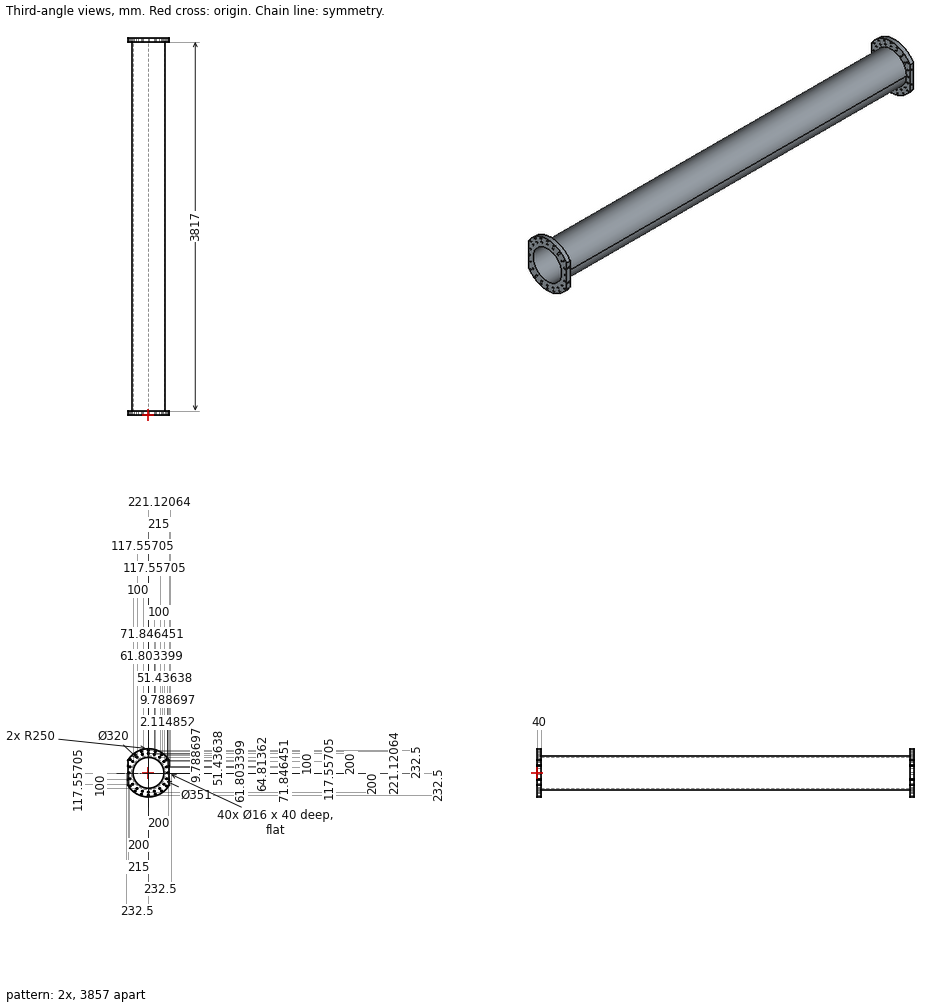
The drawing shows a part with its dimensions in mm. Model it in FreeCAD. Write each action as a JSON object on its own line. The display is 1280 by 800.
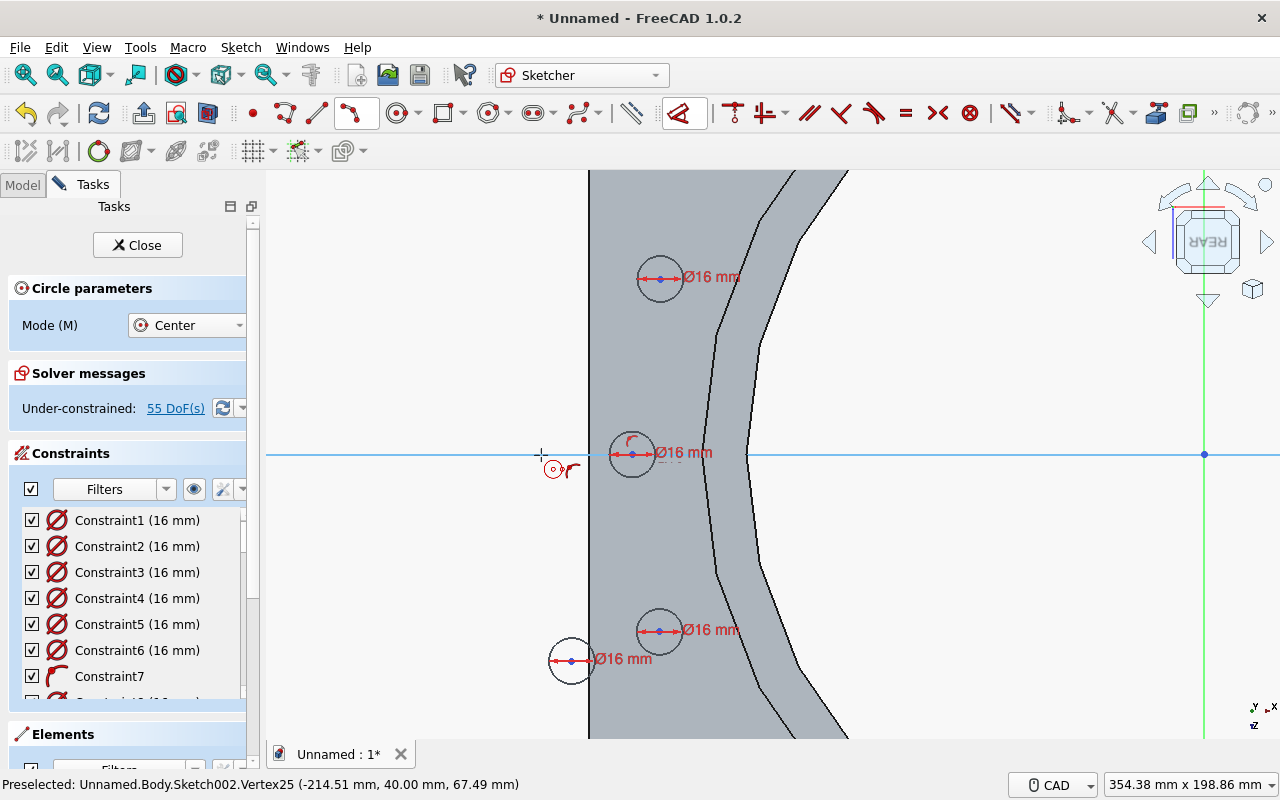
{"action": "left_click", "coordinate": [539, 455]}
{"action": "mouse_move", "coordinate": [555, 438]}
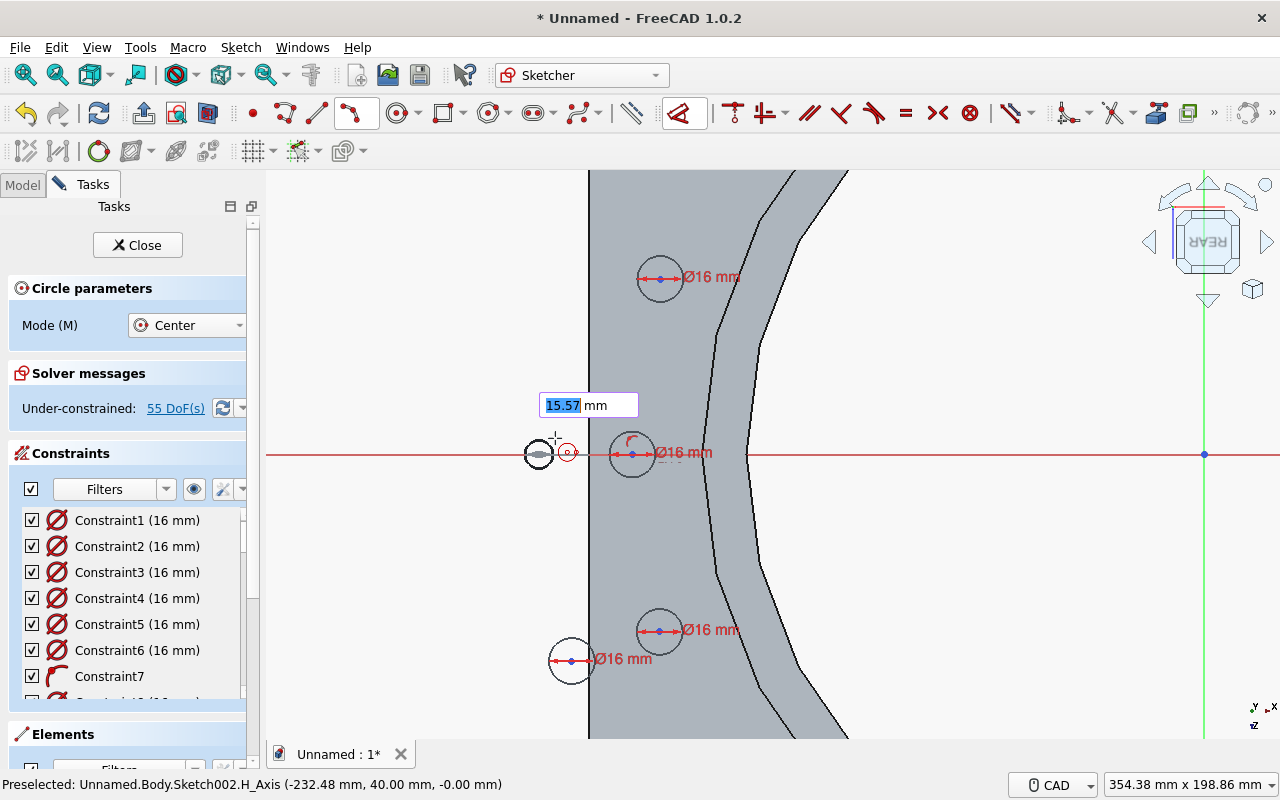
{"action": "type", "text": "16"}
{"action": "key", "text": "Return"}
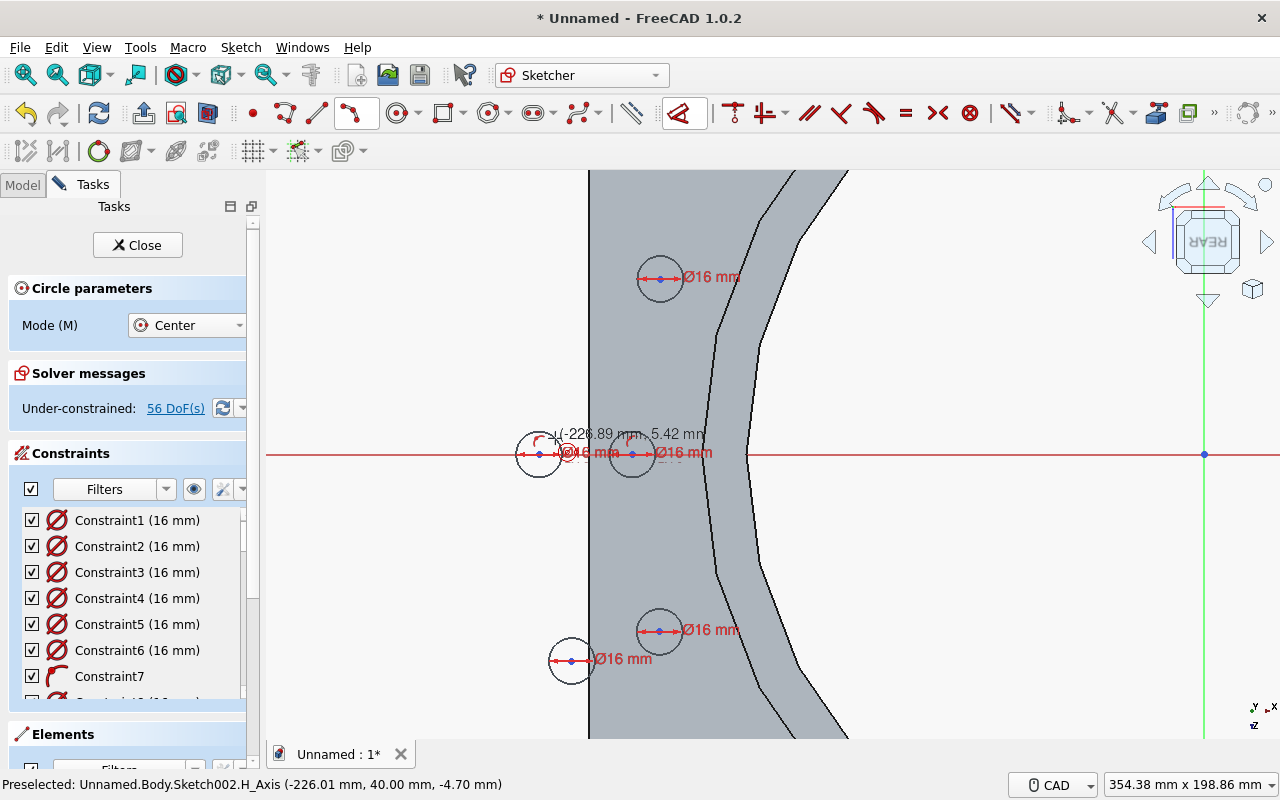
{"action": "left_click", "coordinate": [572, 249]}
{"action": "mouse_move", "coordinate": [588, 233]}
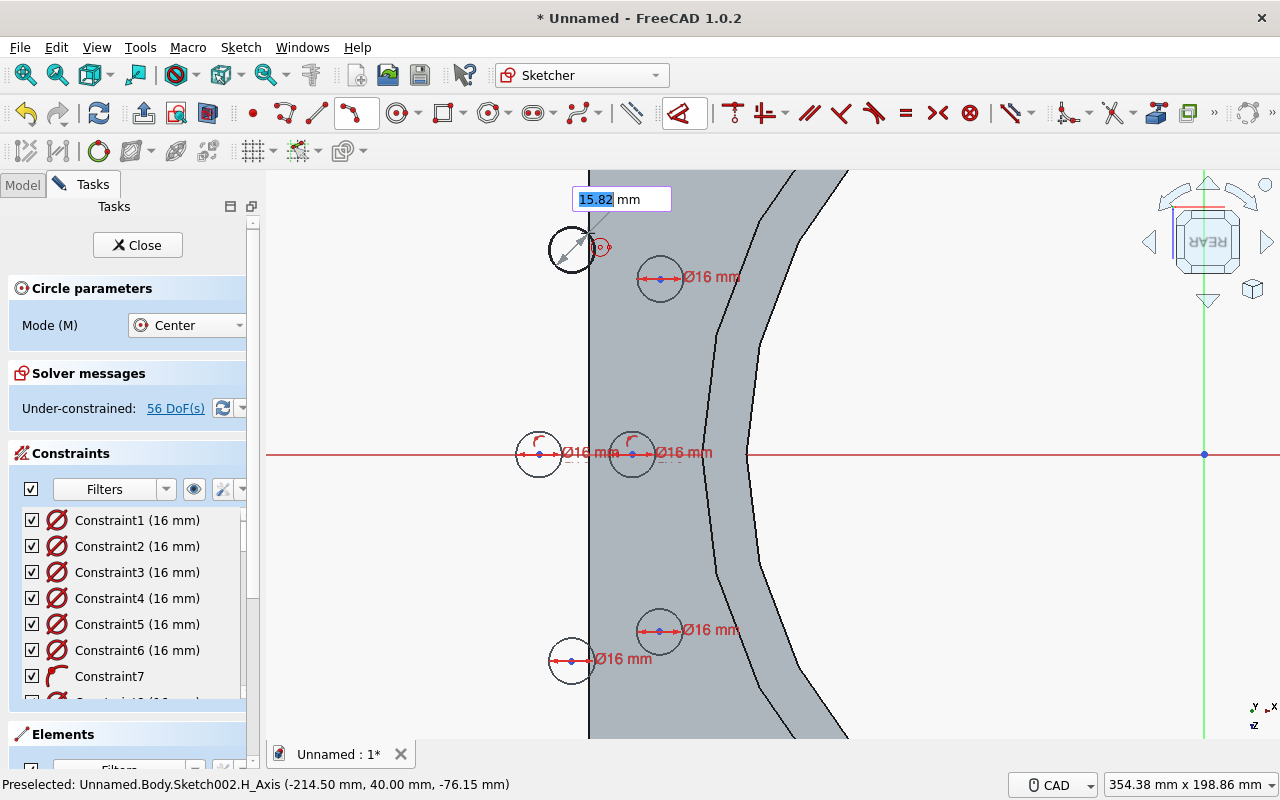
{"action": "type", "text": "16"}
{"action": "key", "text": "Return"}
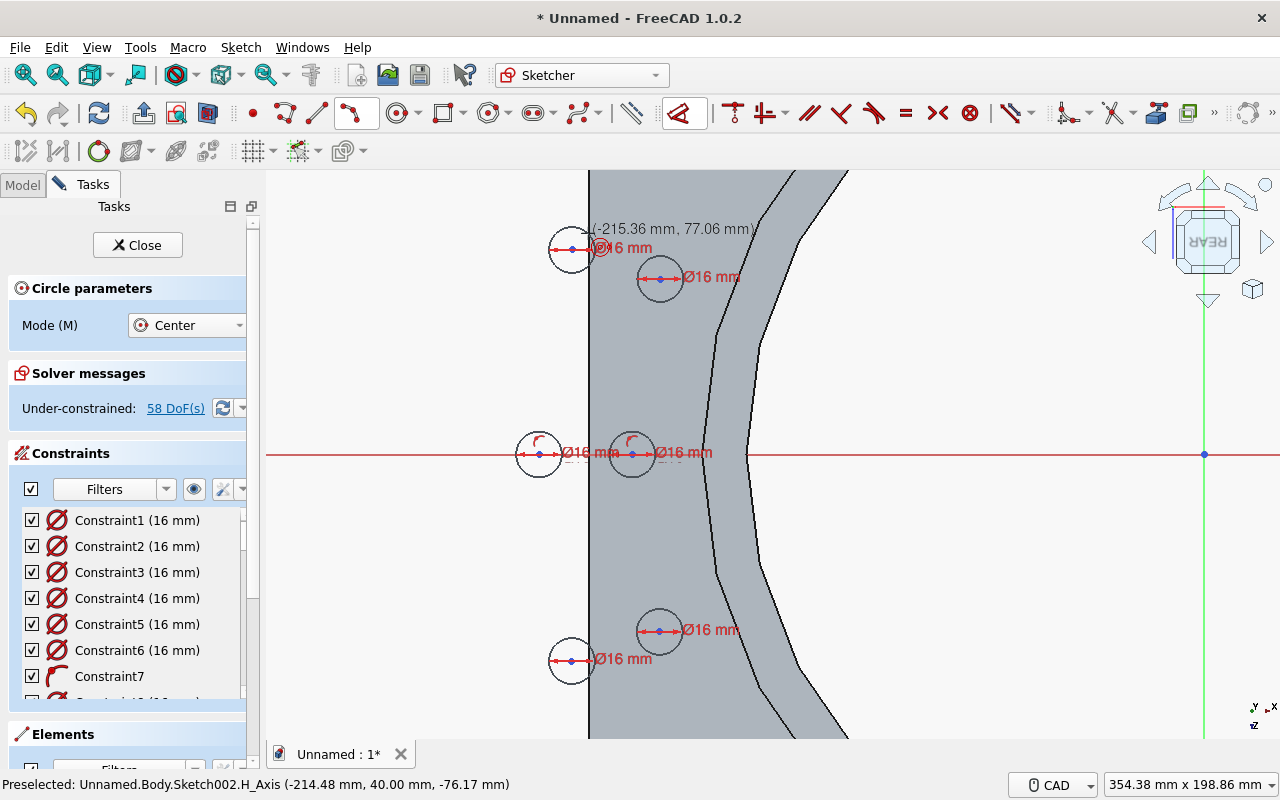
{"action": "scroll", "coordinate": [541, 454], "scroll_direction": "down", "scroll_amount": 7}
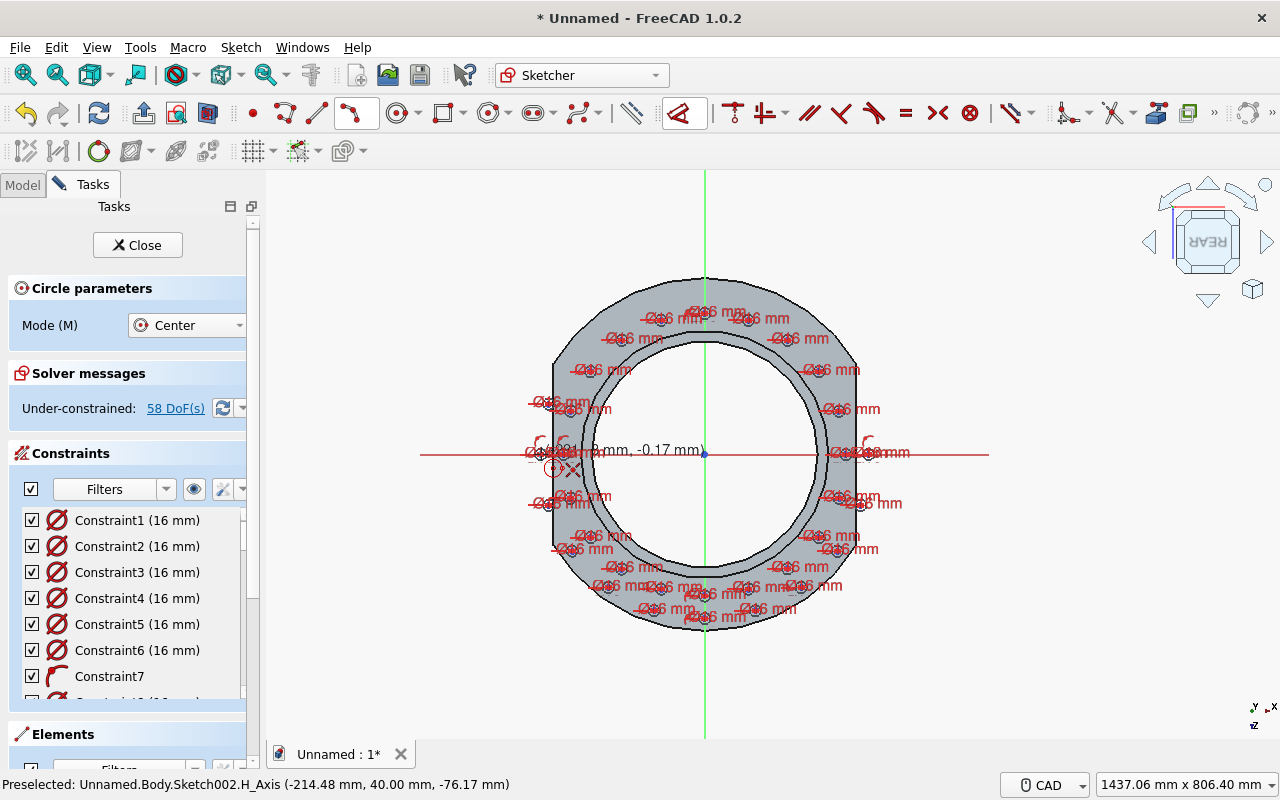
{"action": "scroll", "coordinate": [572, 358], "scroll_direction": "up", "scroll_amount": 7}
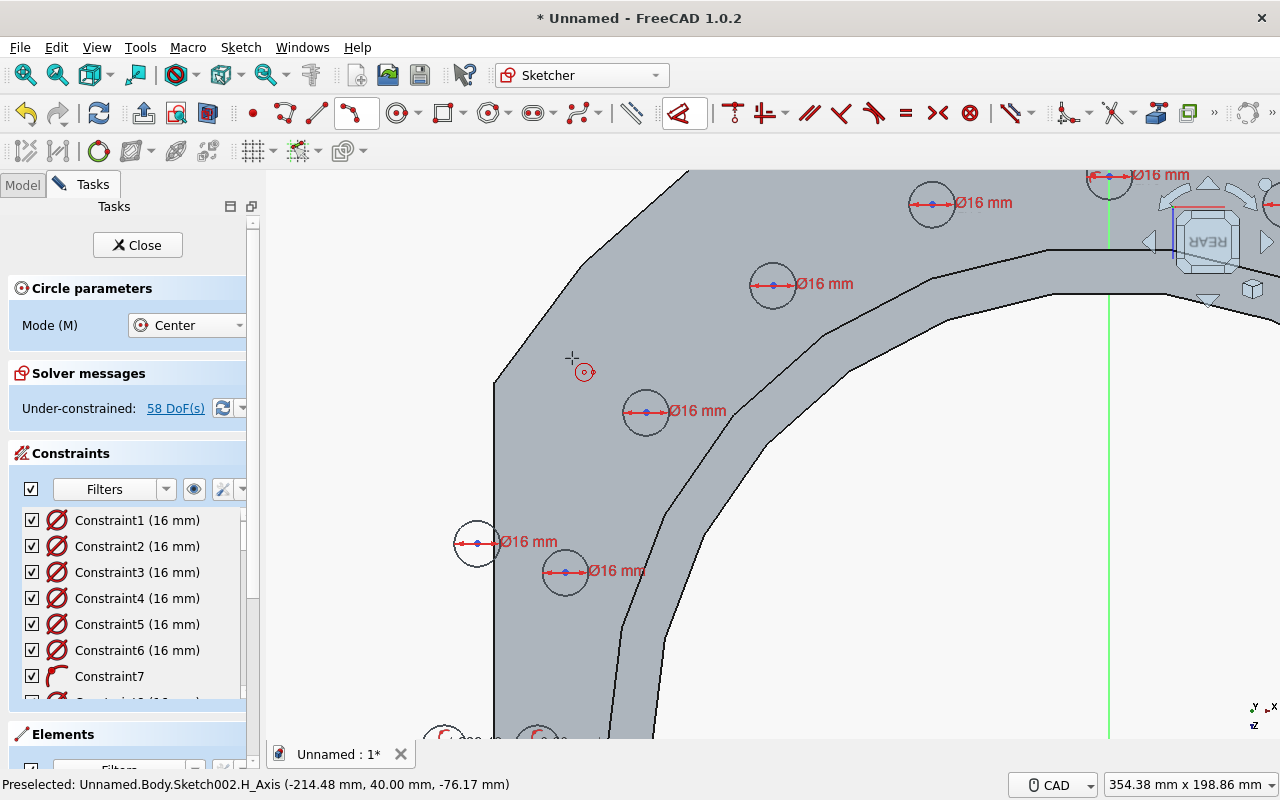
{"action": "left_click", "coordinate": [571, 357]}
{"action": "mouse_move", "coordinate": [587, 341]}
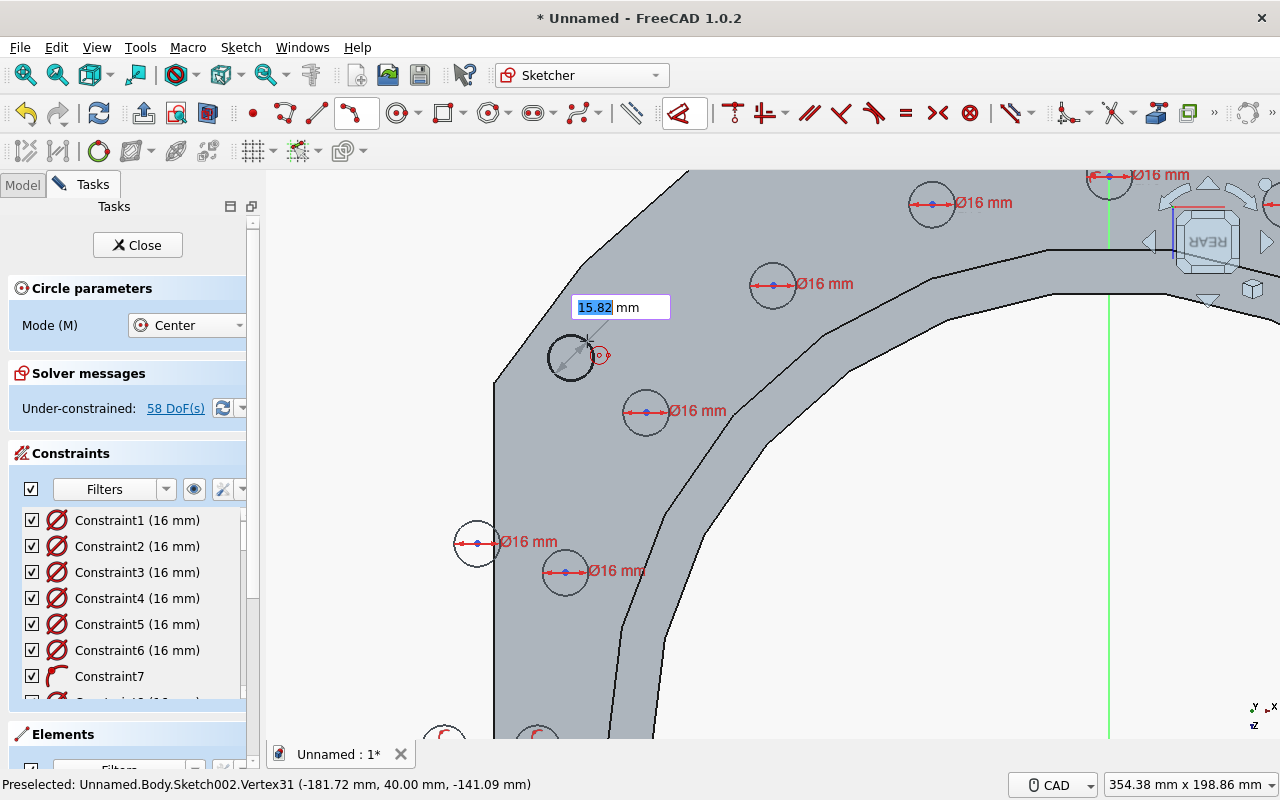
{"action": "type", "text": "16"}
{"action": "key", "text": "Return"}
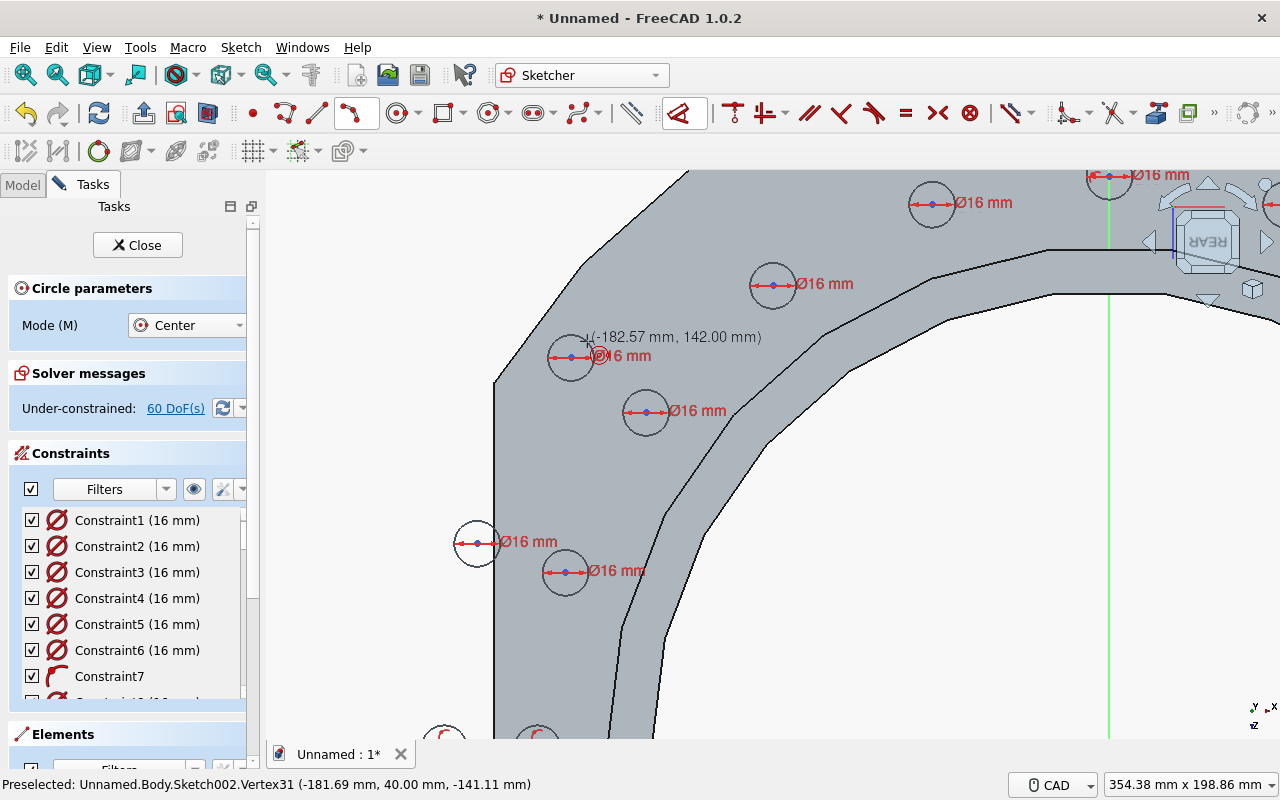
{"action": "left_click", "coordinate": [718, 210]}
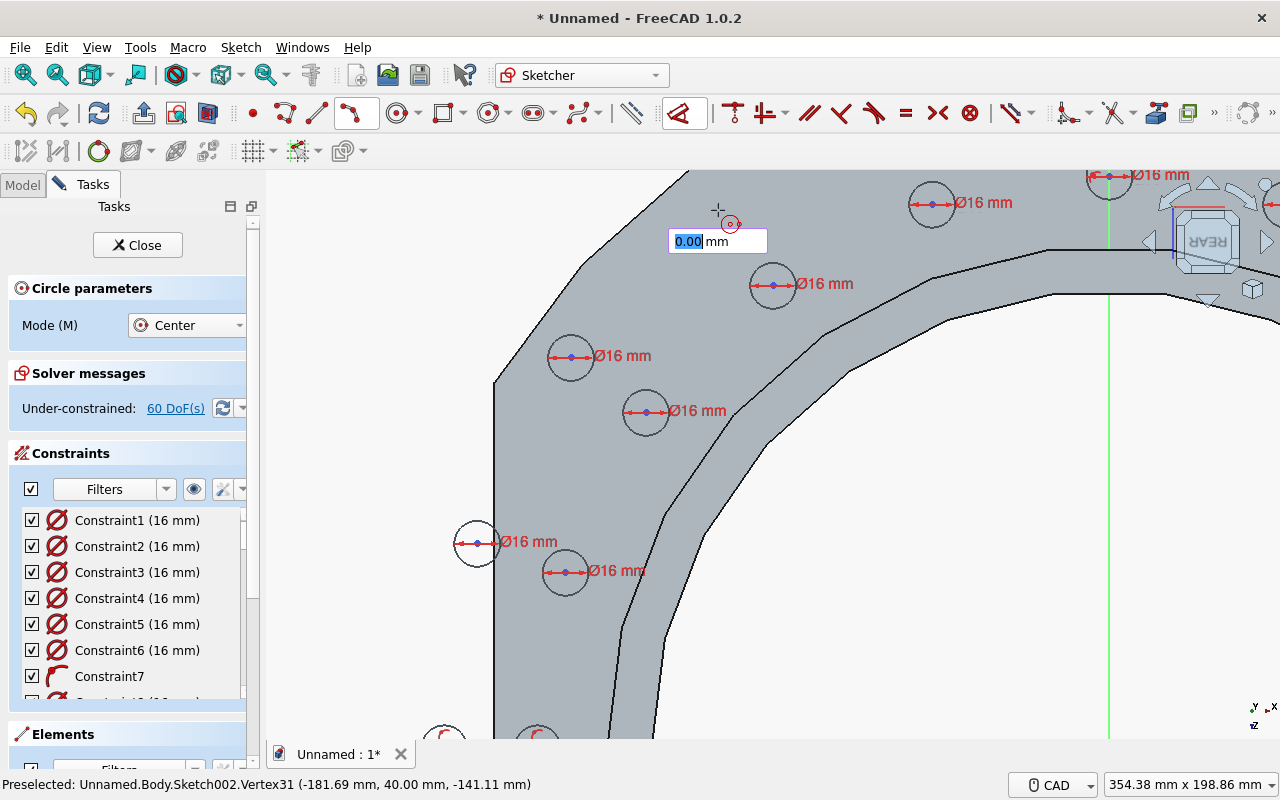
{"action": "scroll", "coordinate": [572, 358], "scroll_direction": "down", "scroll_amount": 7}
{"action": "mouse_move", "coordinate": [612, 318]}